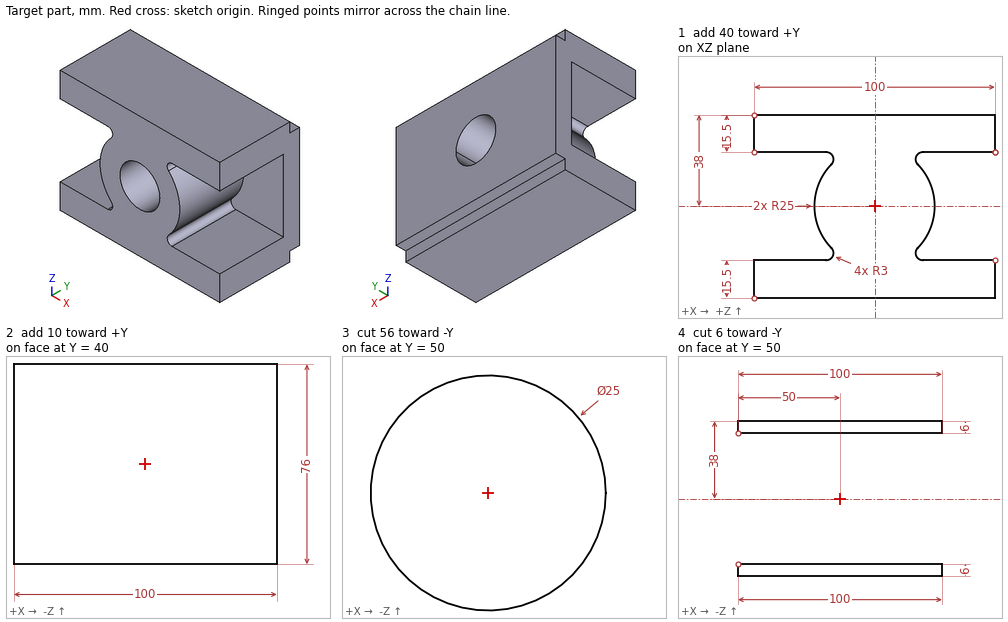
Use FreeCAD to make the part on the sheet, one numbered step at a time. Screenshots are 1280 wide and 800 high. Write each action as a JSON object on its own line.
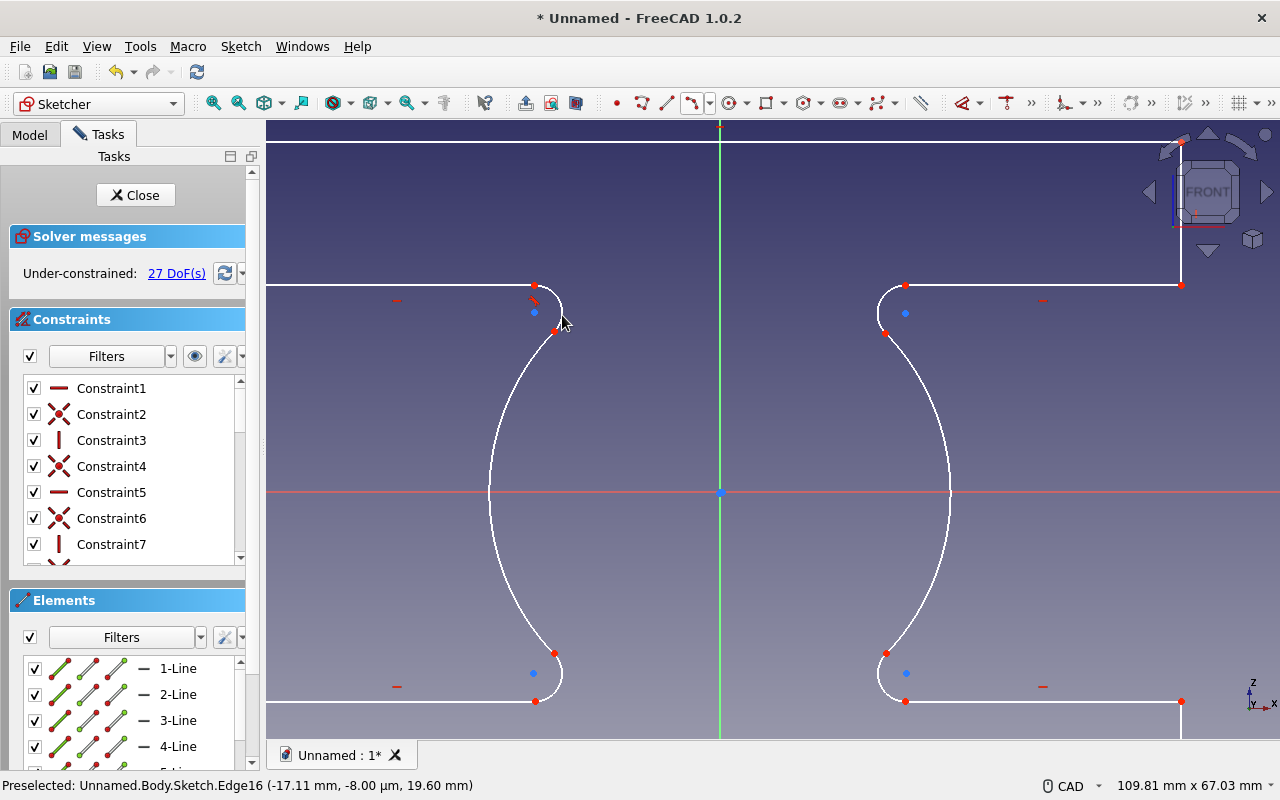
{"action": "left_click", "coordinate": [1098, 285]}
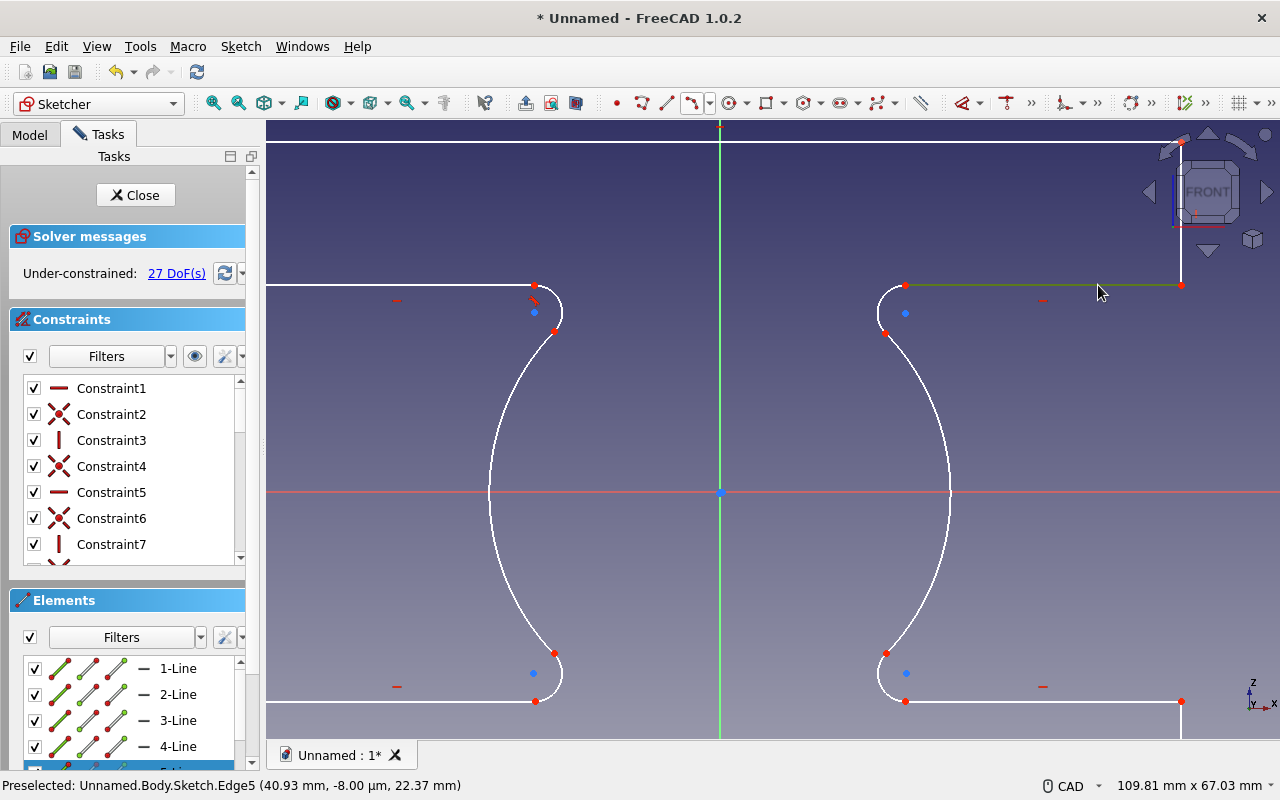
{"action": "left_click", "coordinate": [887, 292]}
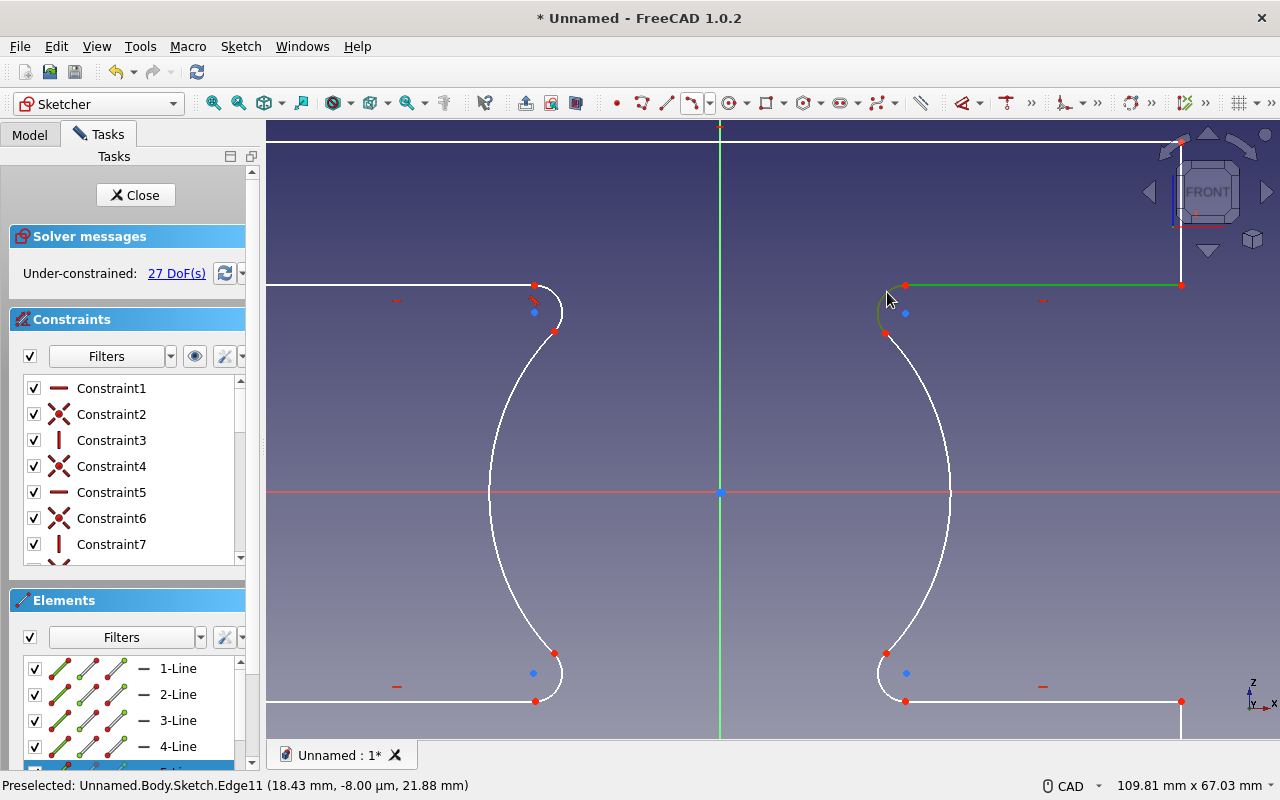
{"action": "key", "text": "t"}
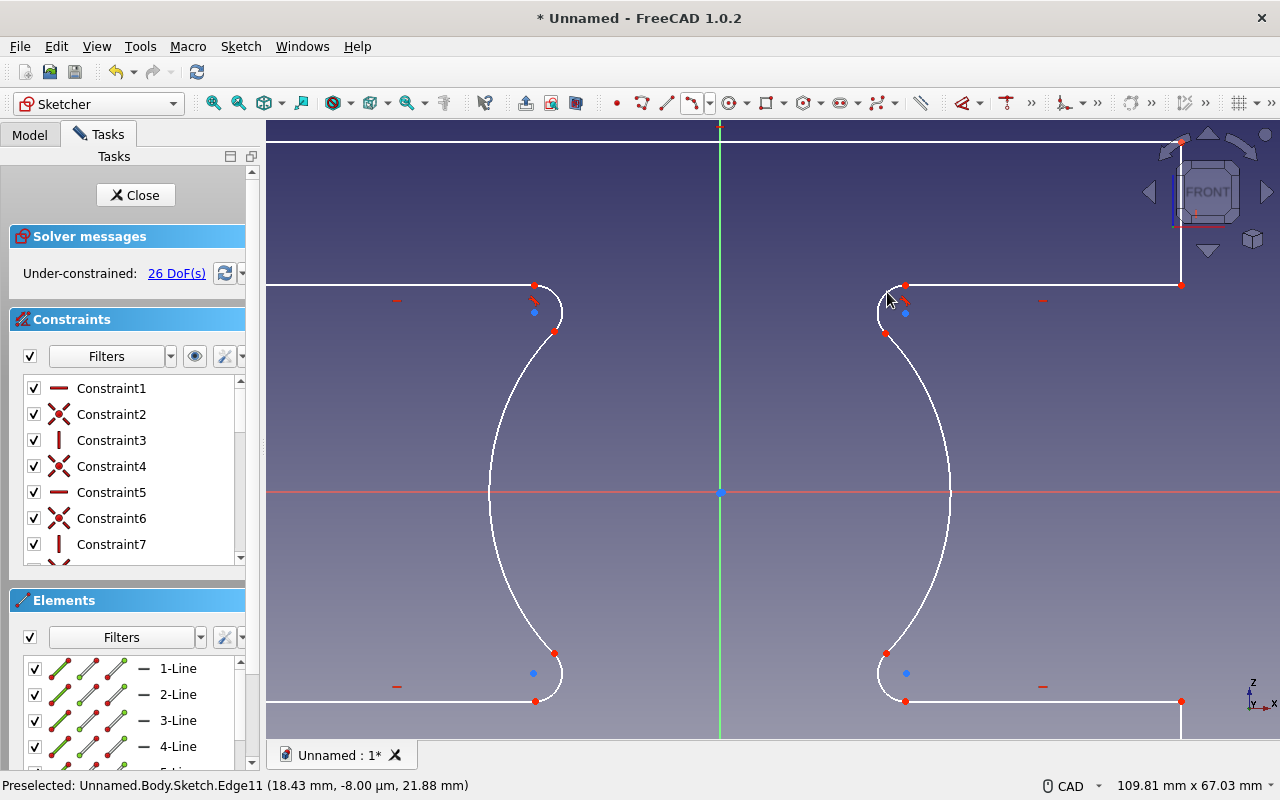
{"action": "left_click", "coordinate": [988, 702]}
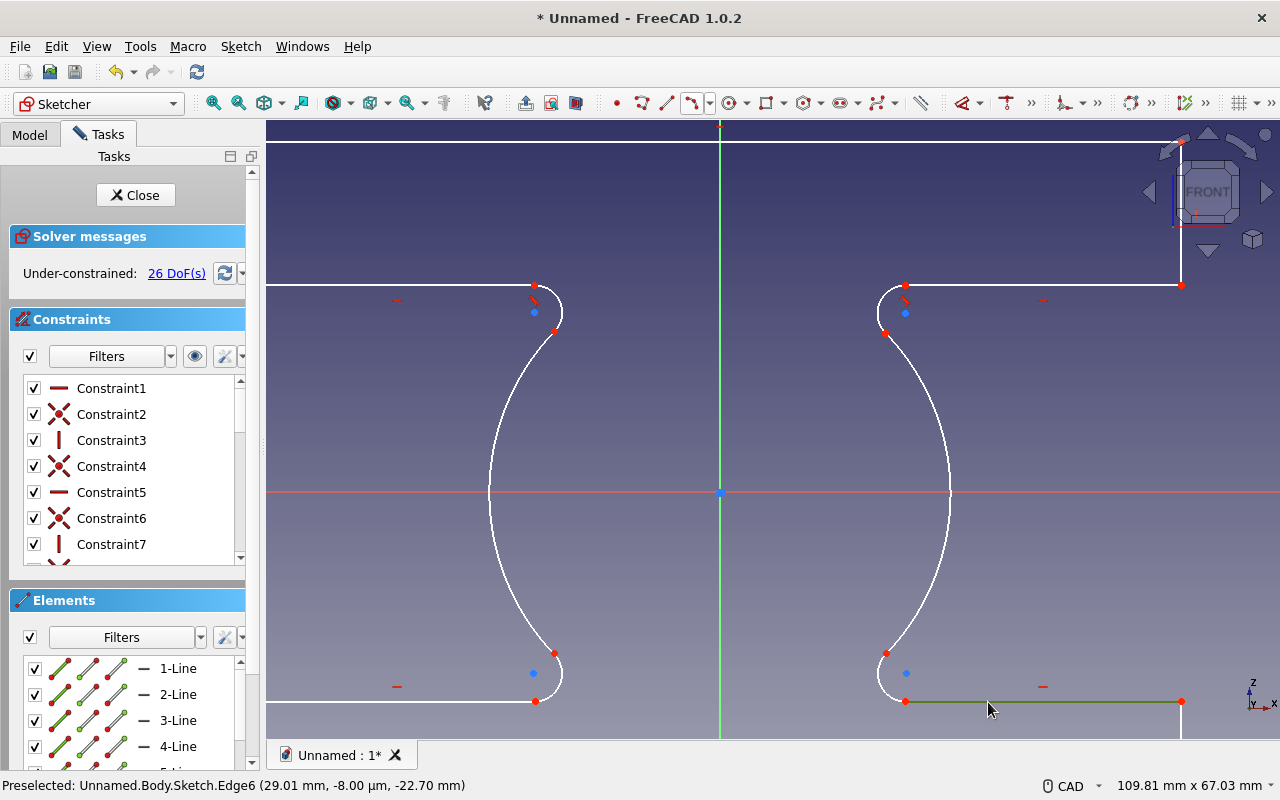
{"action": "left_click", "coordinate": [878, 671]}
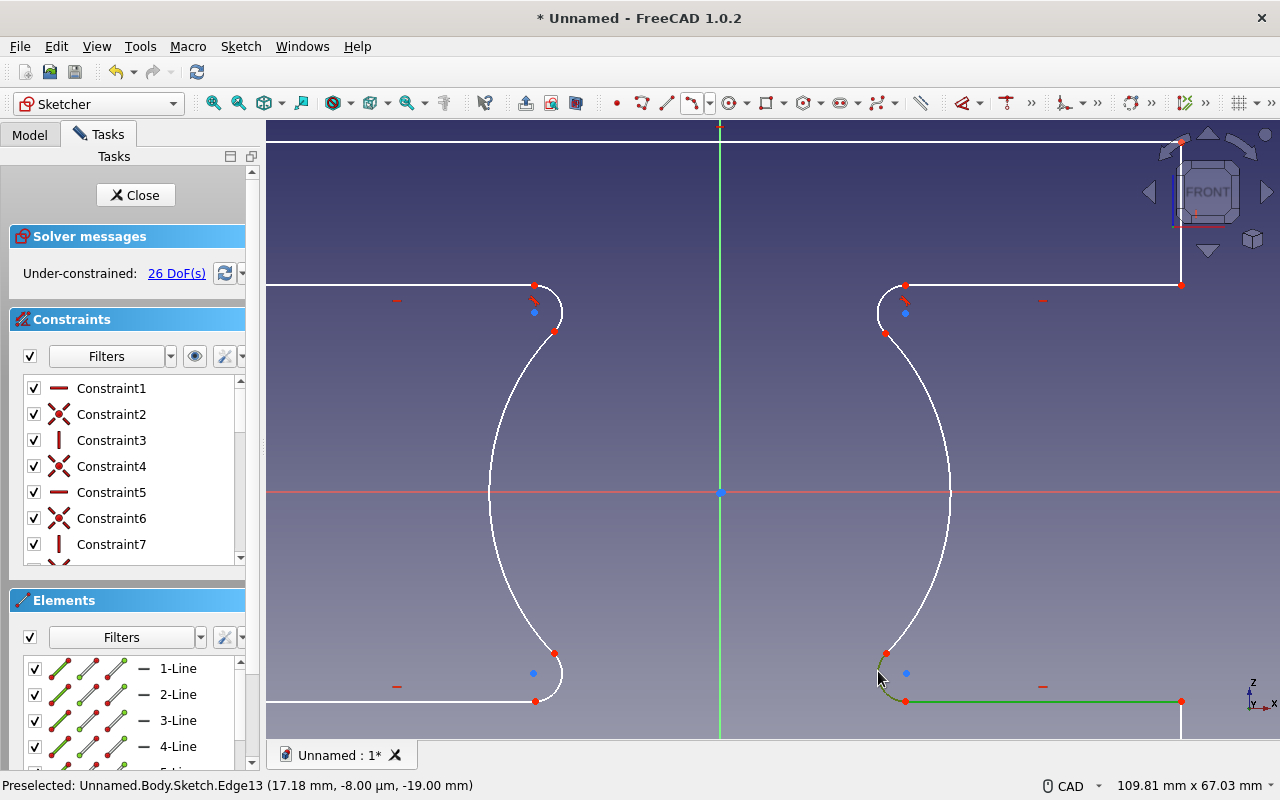
{"action": "key", "text": "t"}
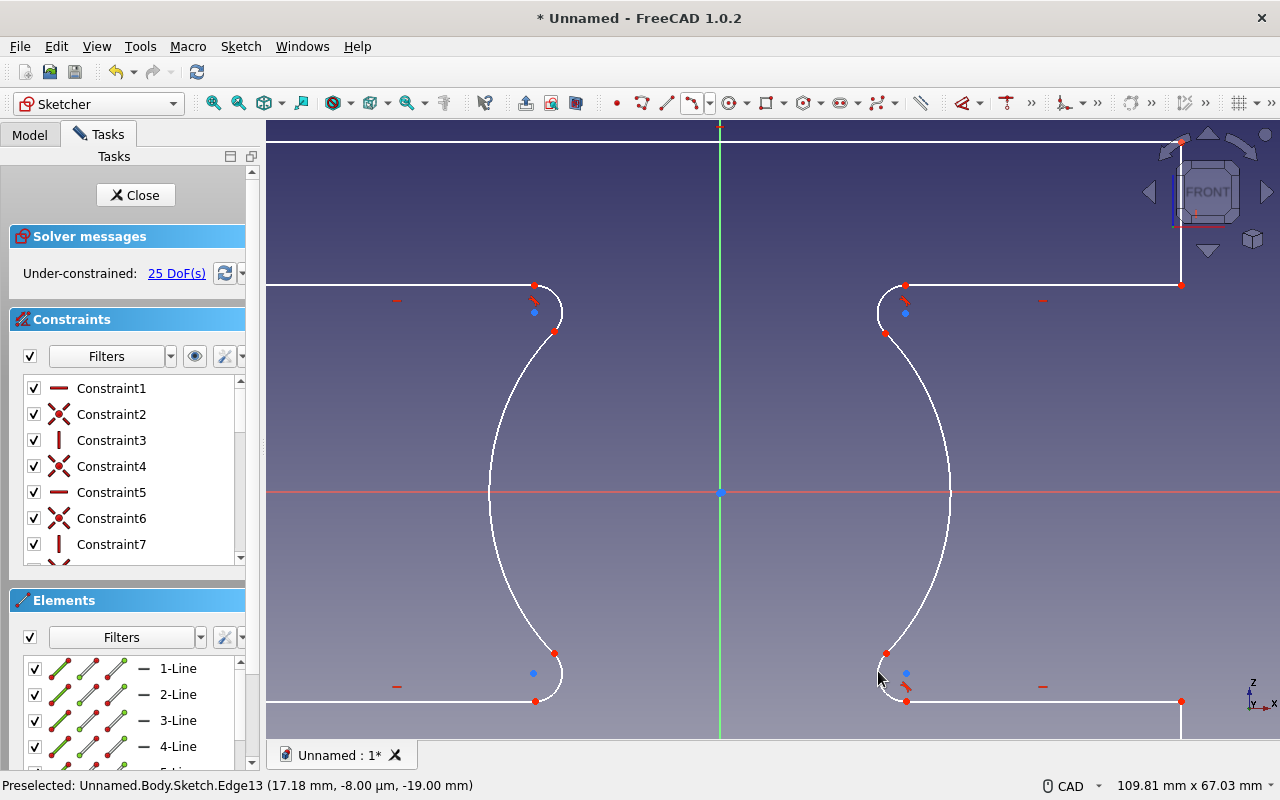
{"action": "left_click", "coordinate": [342, 702]}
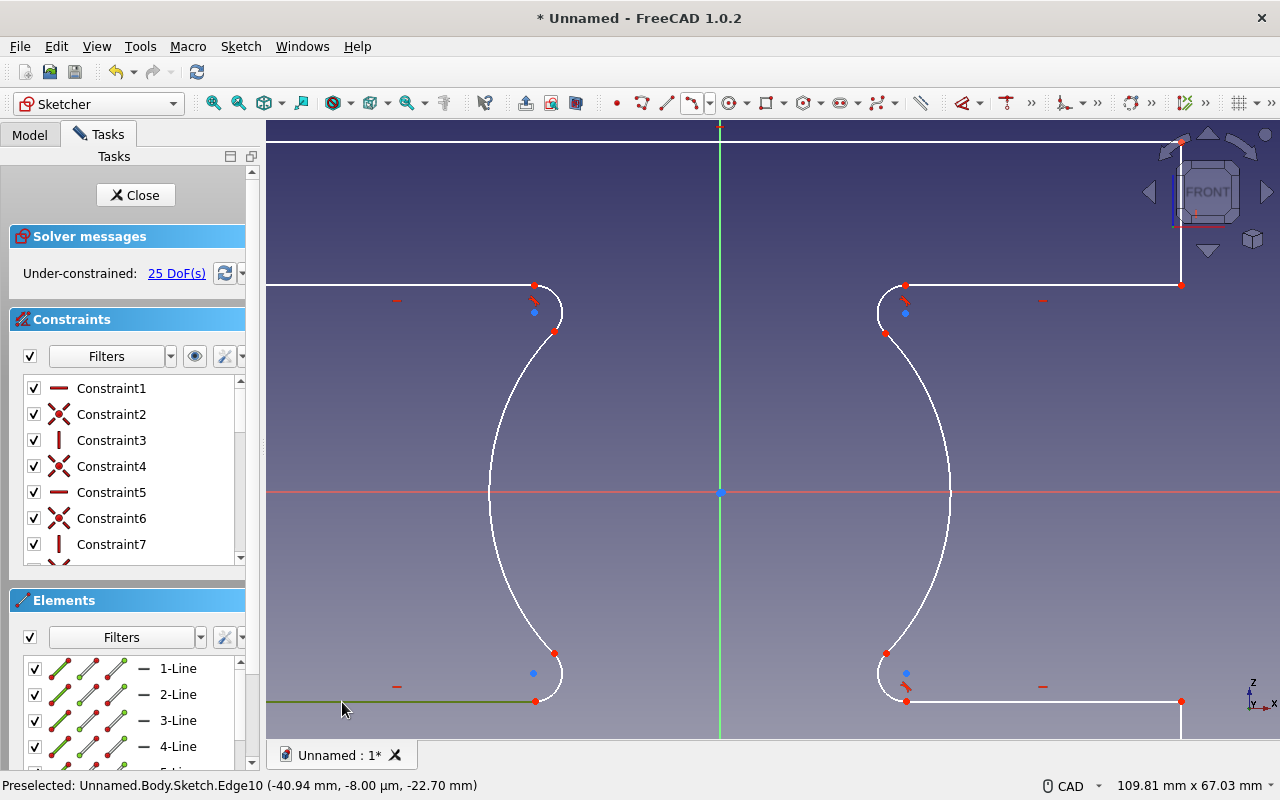
{"action": "left_click", "coordinate": [553, 694]}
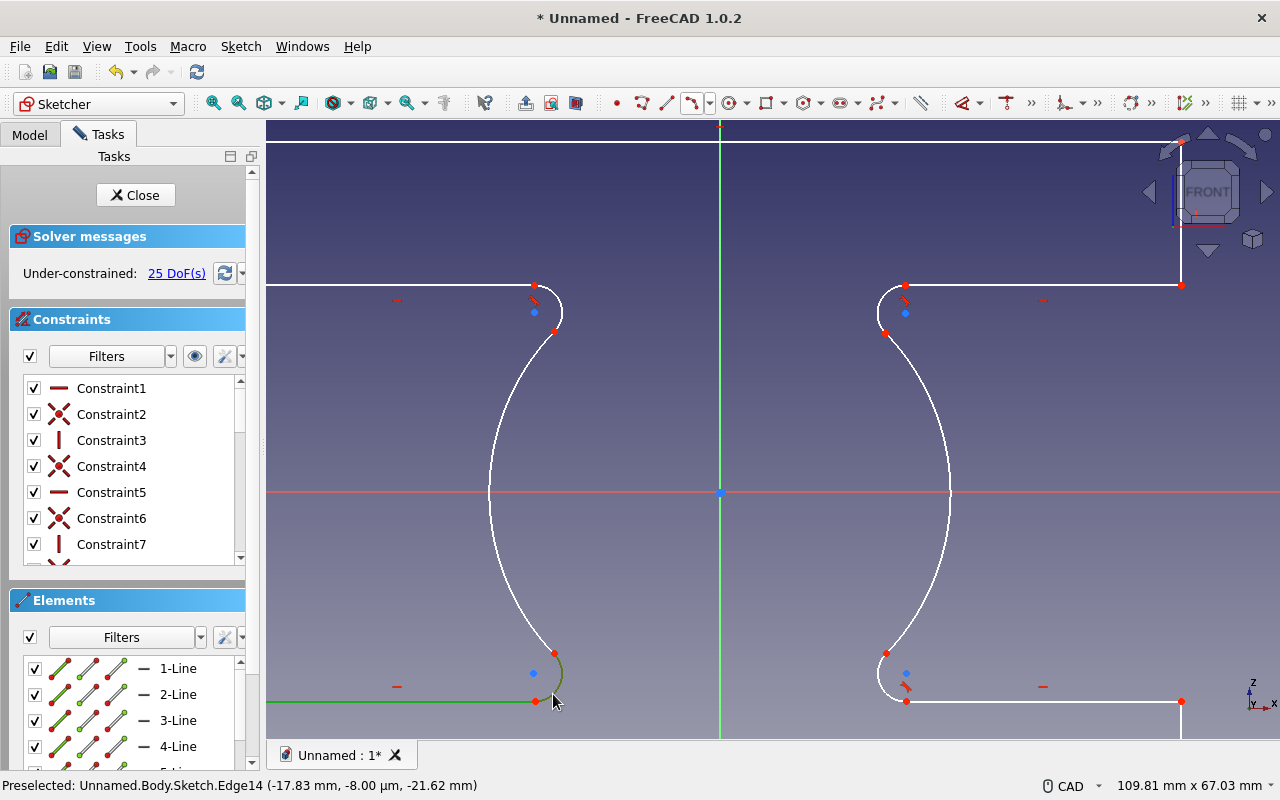
{"action": "key", "text": "t"}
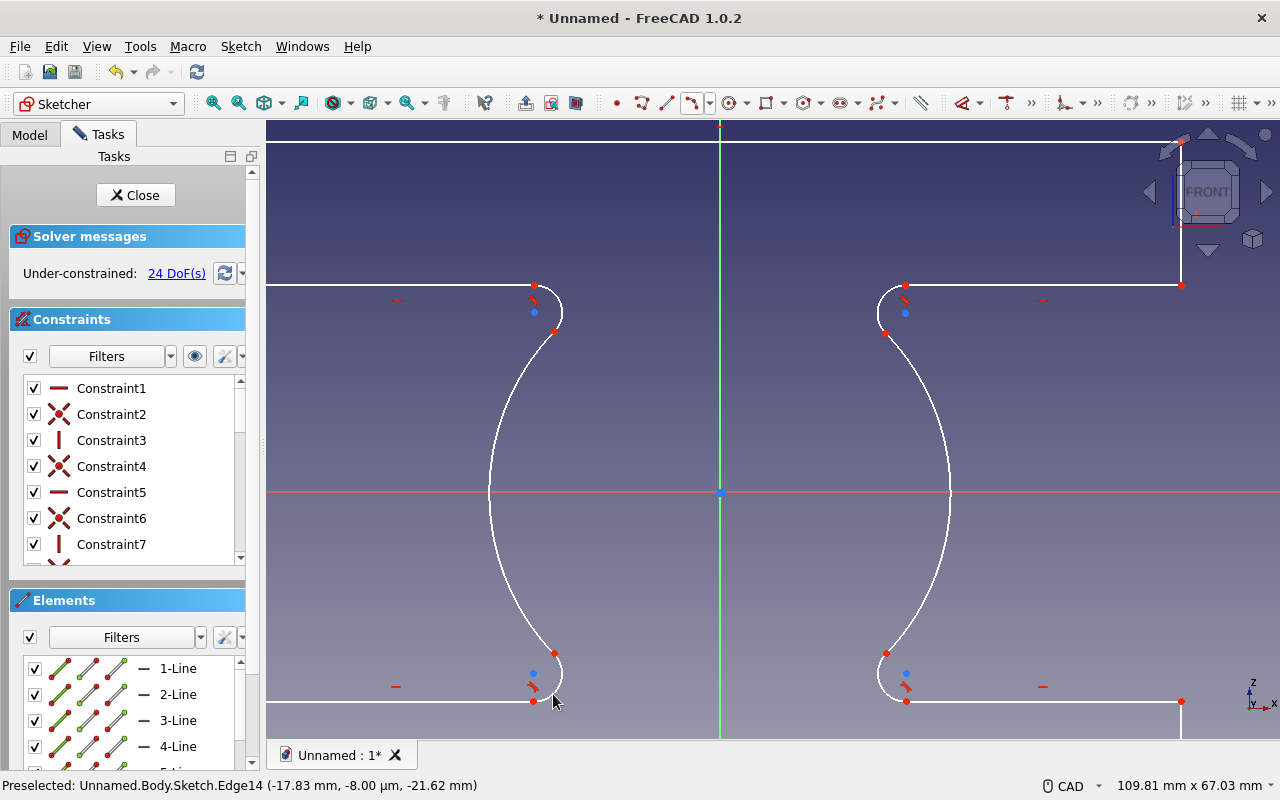
{"action": "left_click", "coordinate": [887, 292]}